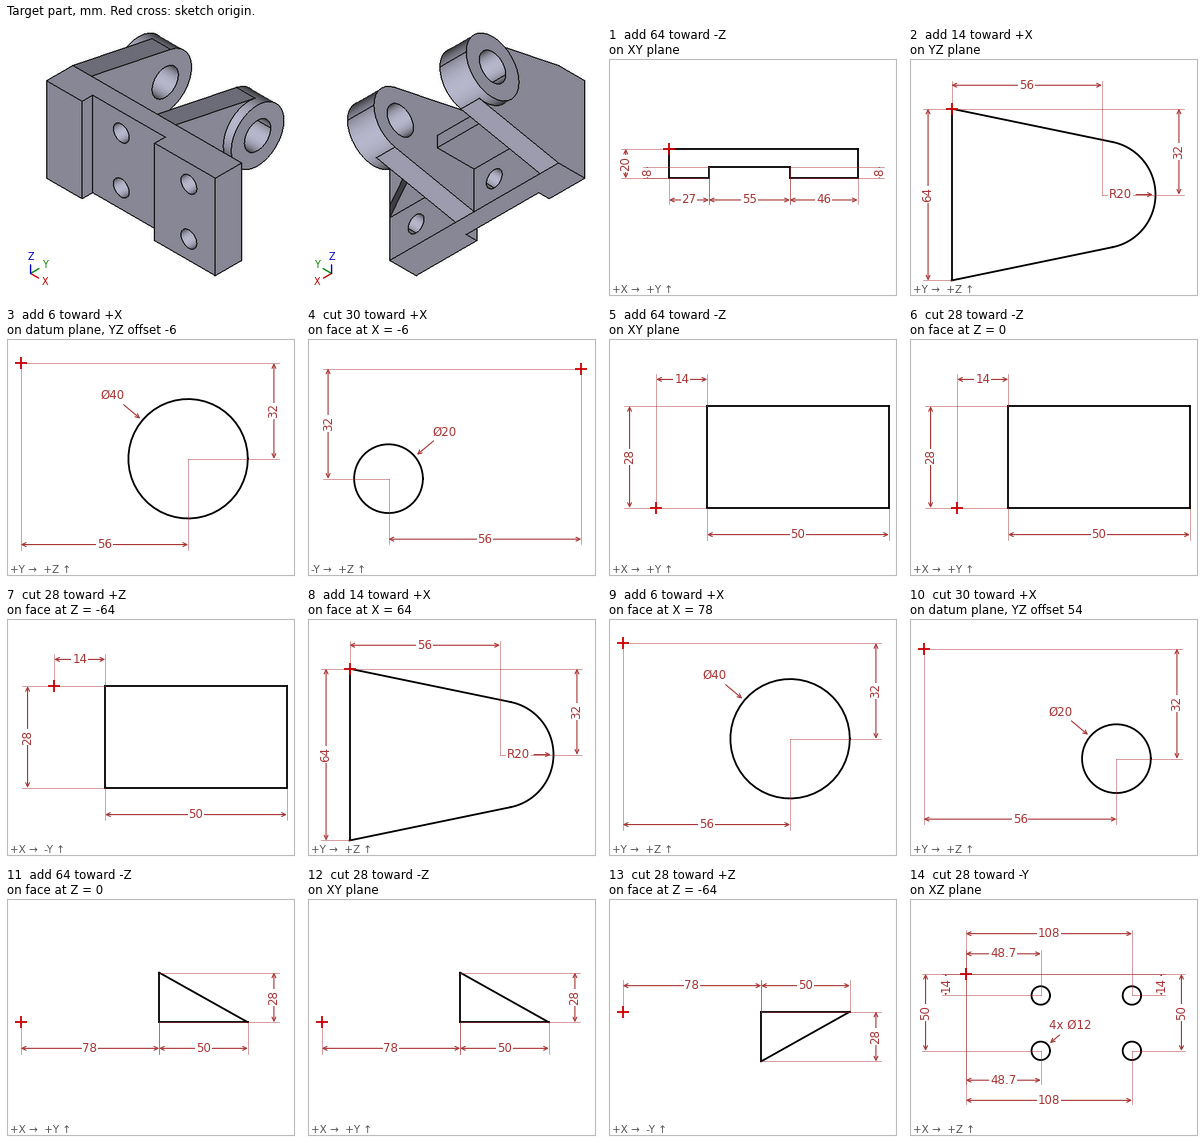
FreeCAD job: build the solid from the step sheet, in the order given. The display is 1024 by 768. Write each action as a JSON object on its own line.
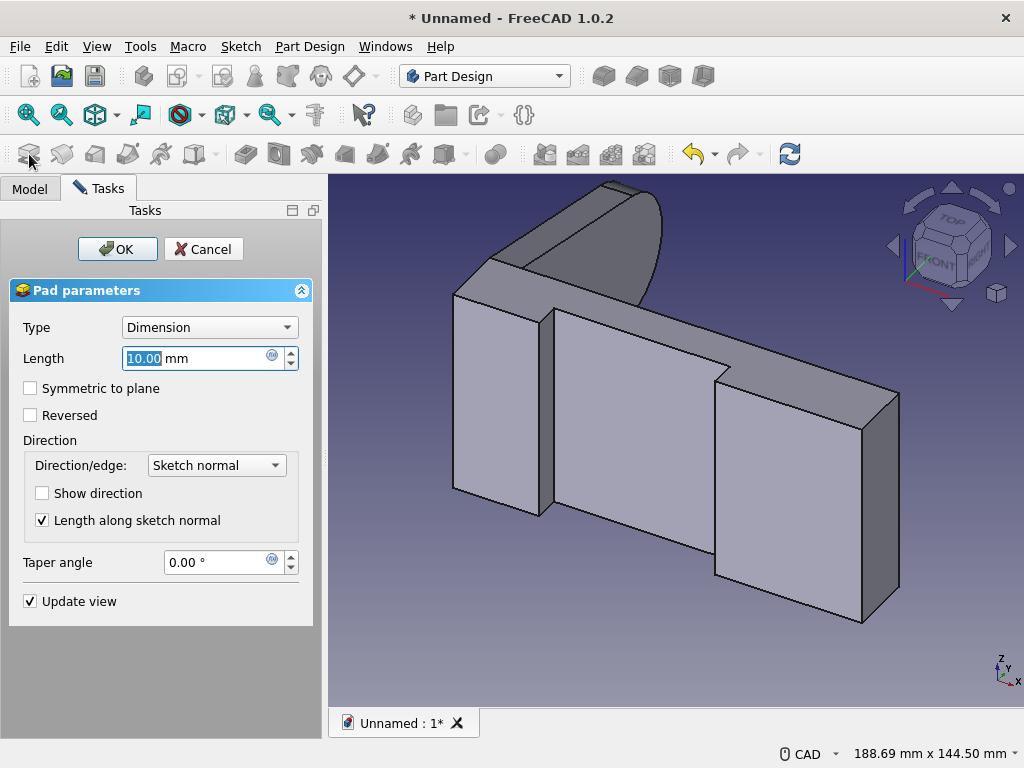
{"action": "type", "text": "14"}
{"action": "key", "text": "Tab"}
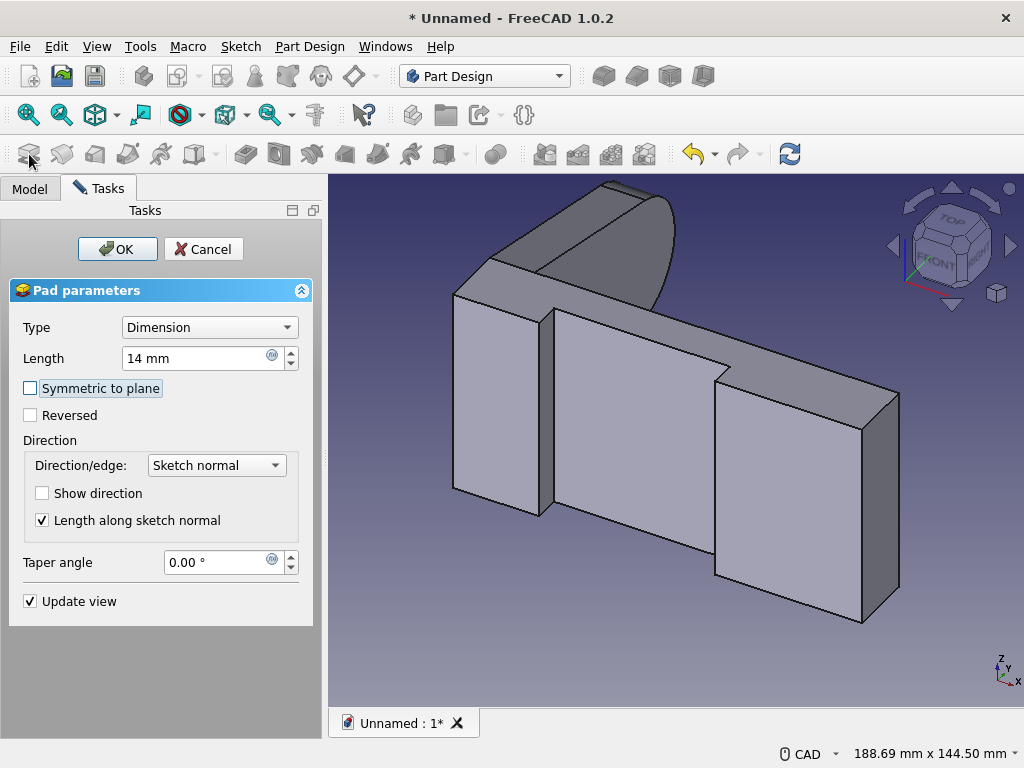
{"action": "left_click", "coordinate": [118, 249]}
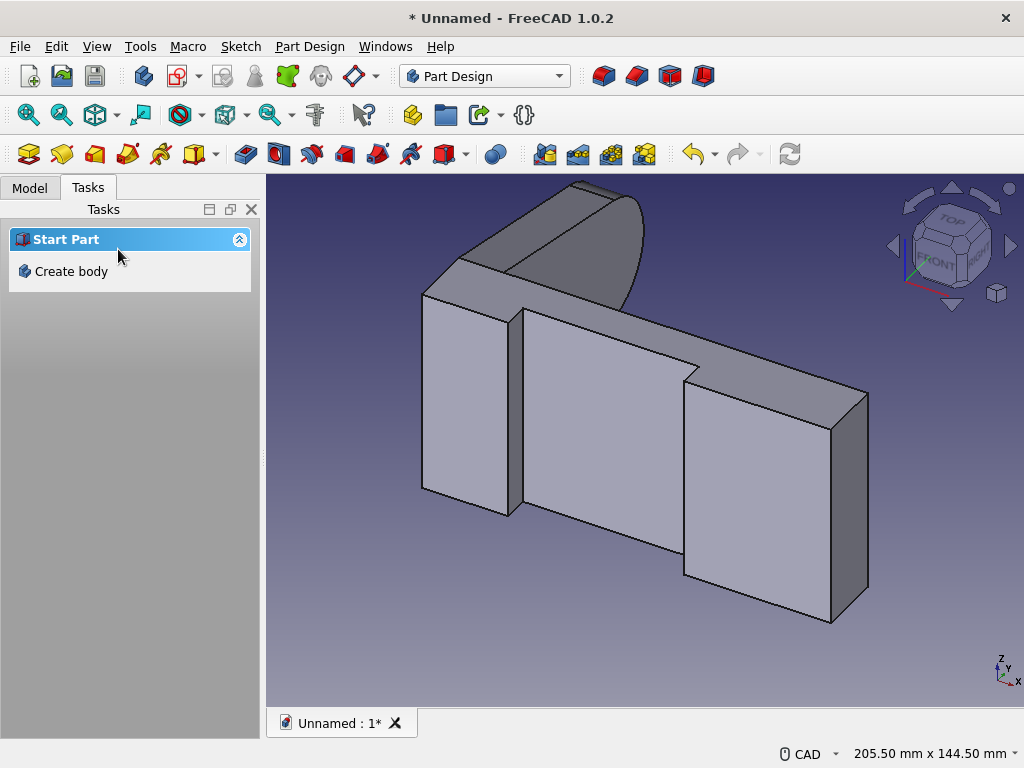
{"action": "left_click", "coordinate": [29, 116]}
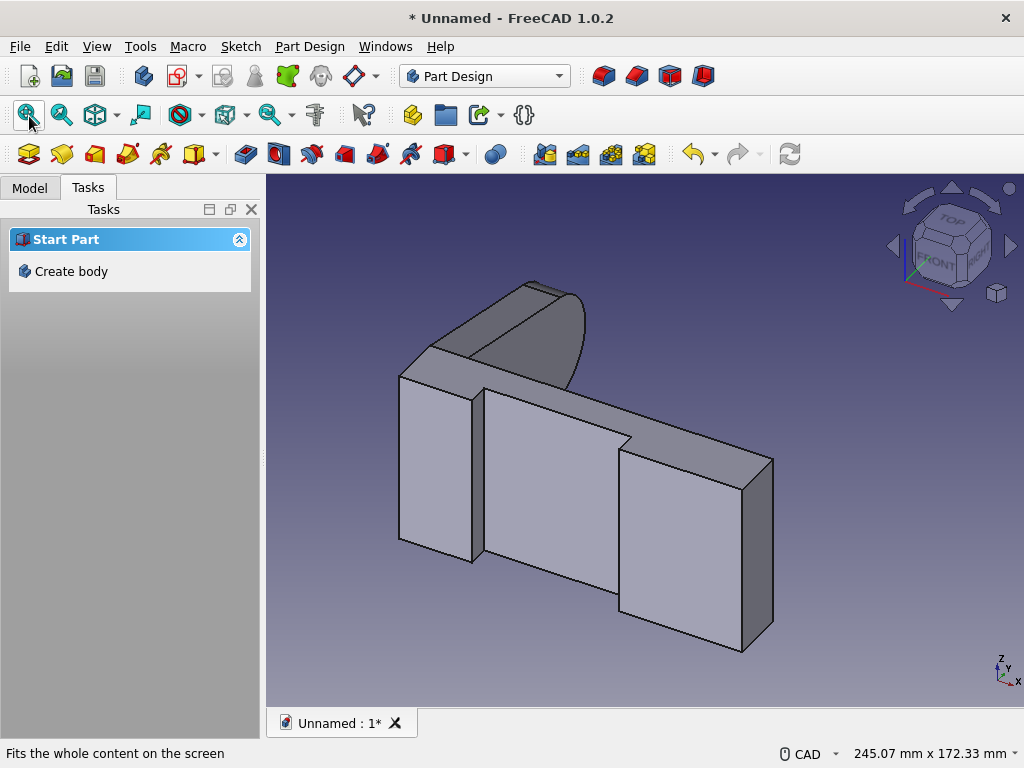
{"action": "left_click", "coordinate": [30, 188]}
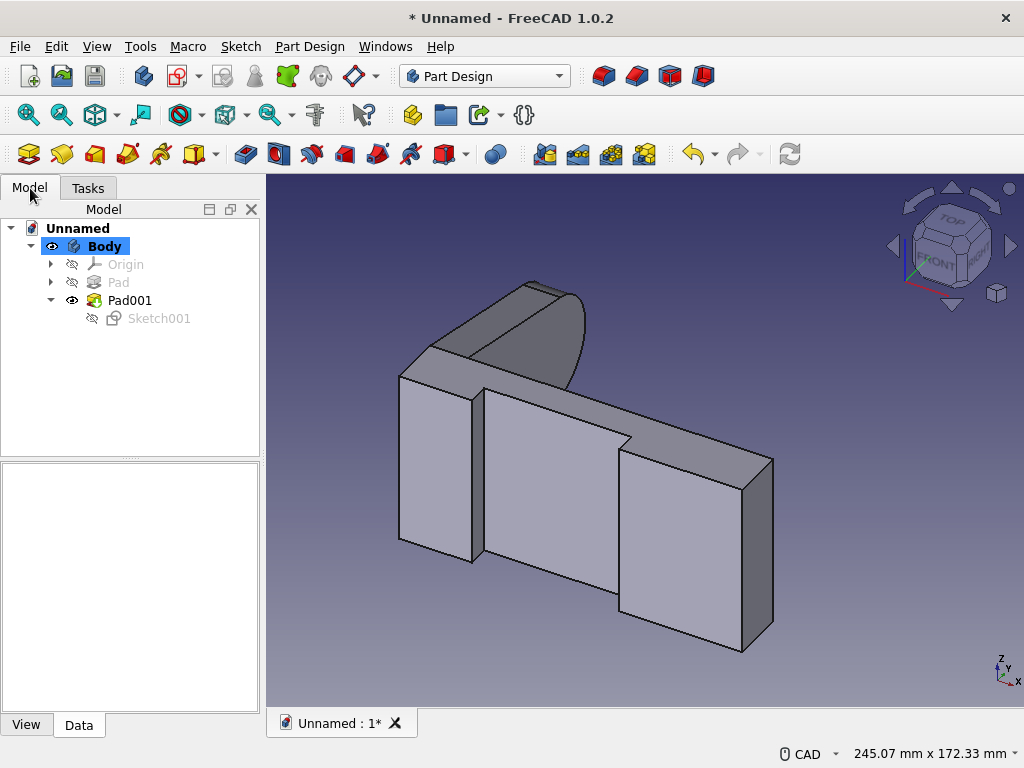
{"action": "left_click", "coordinate": [51, 264]}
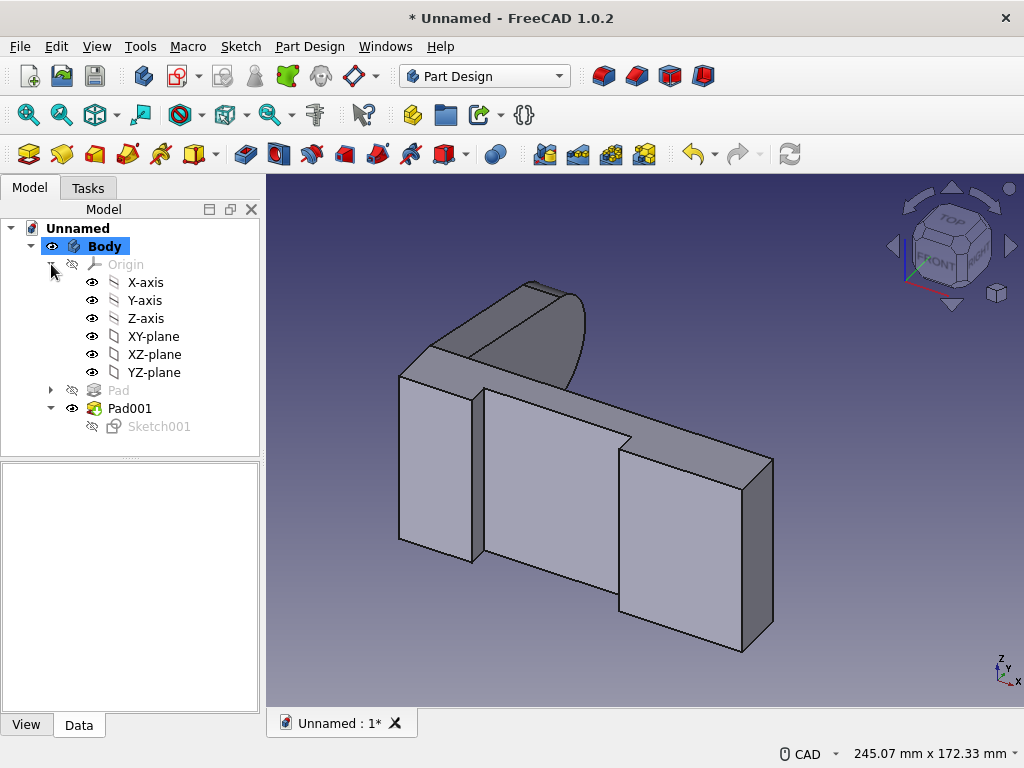
{"action": "left_click", "coordinate": [137, 372]}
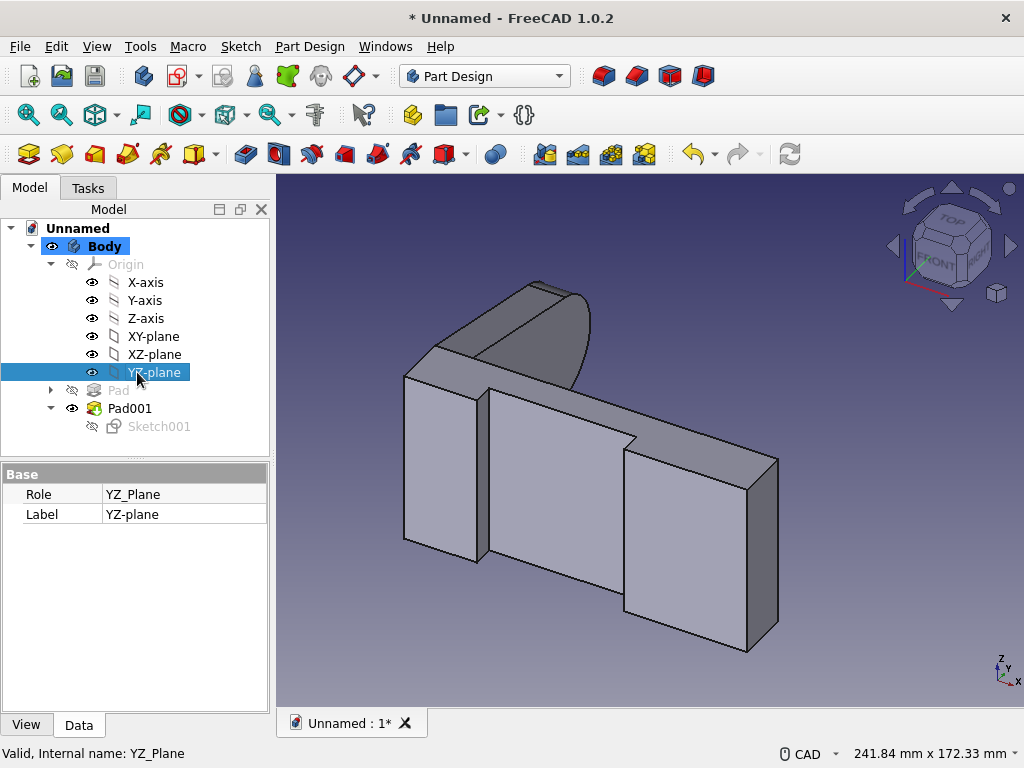
{"action": "left_click", "coordinate": [354, 76]}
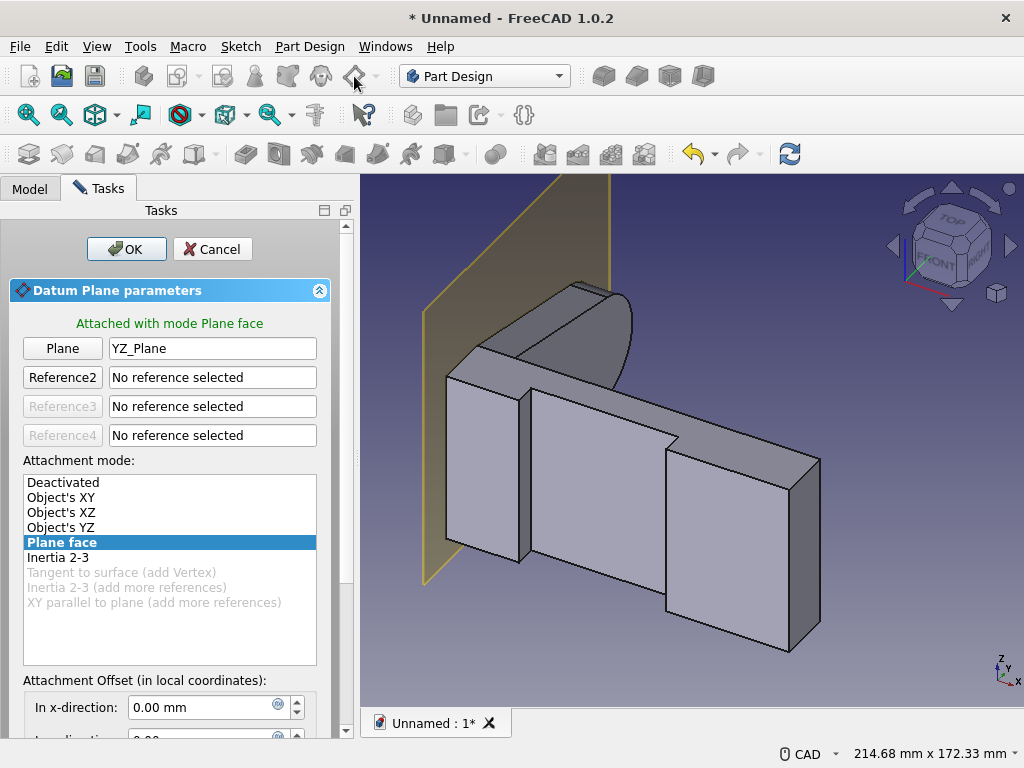
{"action": "scroll", "coordinate": [346, 479], "scroll_direction": "down", "scroll_amount": 2}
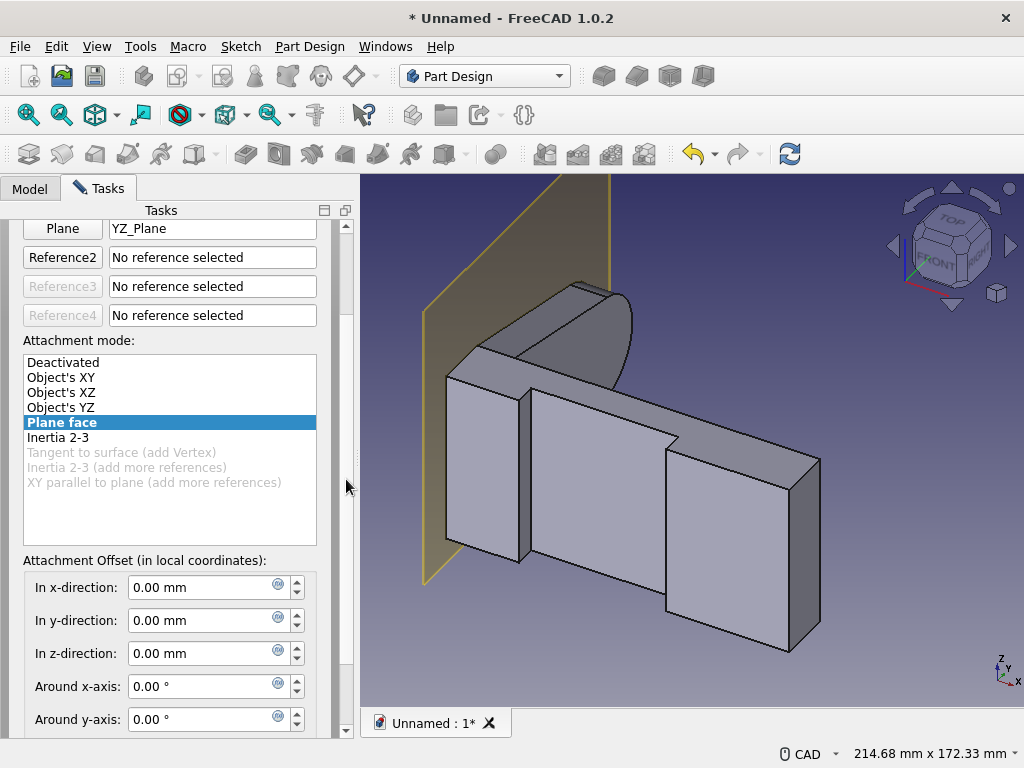
{"action": "triple_click", "coordinate": [210, 654]}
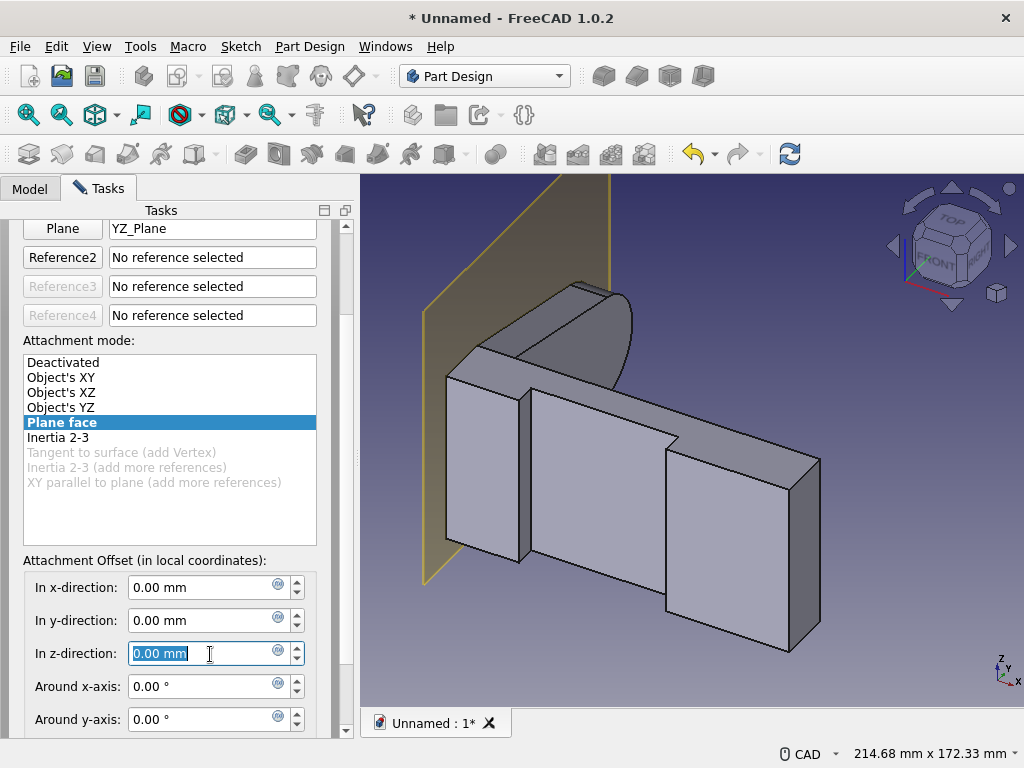
{"action": "type", "text": "-6"}
{"action": "key", "text": "Tab"}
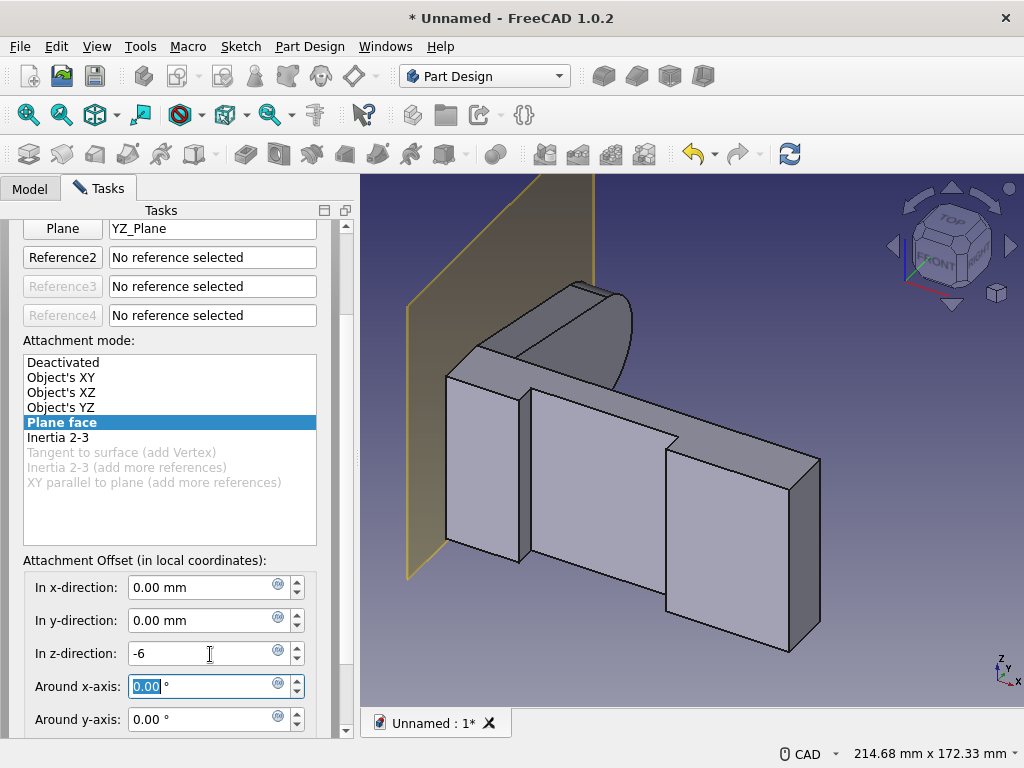
{"action": "scroll", "coordinate": [346, 479], "scroll_direction": "up", "scroll_amount": 3}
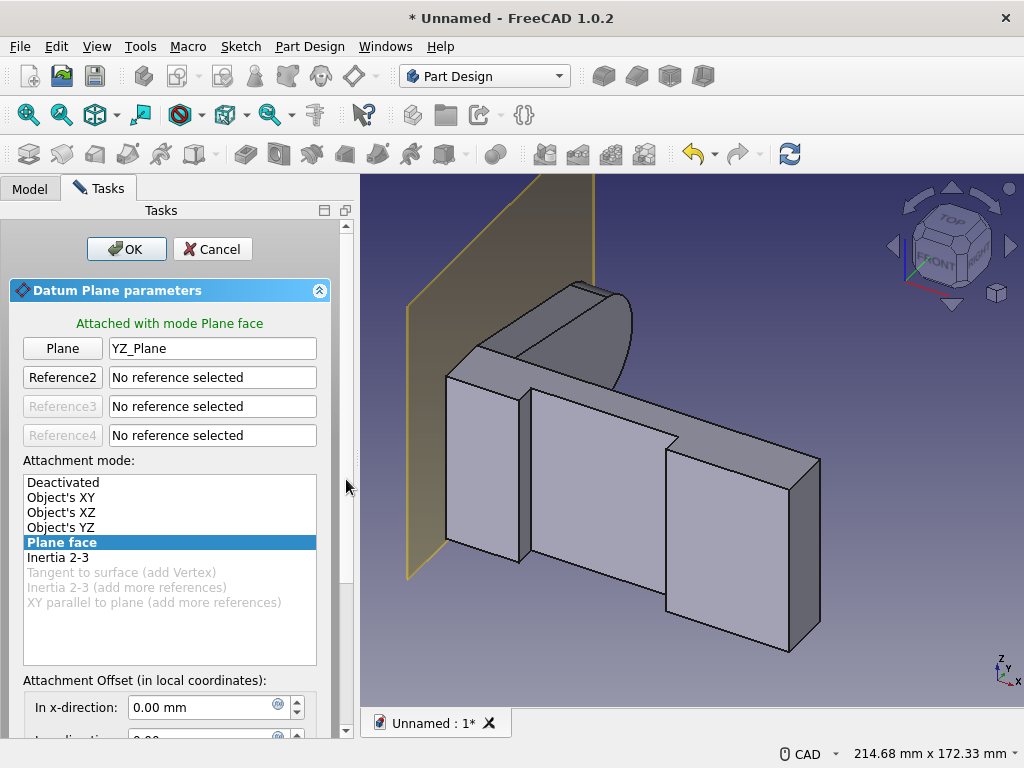
{"action": "left_click", "coordinate": [127, 249]}